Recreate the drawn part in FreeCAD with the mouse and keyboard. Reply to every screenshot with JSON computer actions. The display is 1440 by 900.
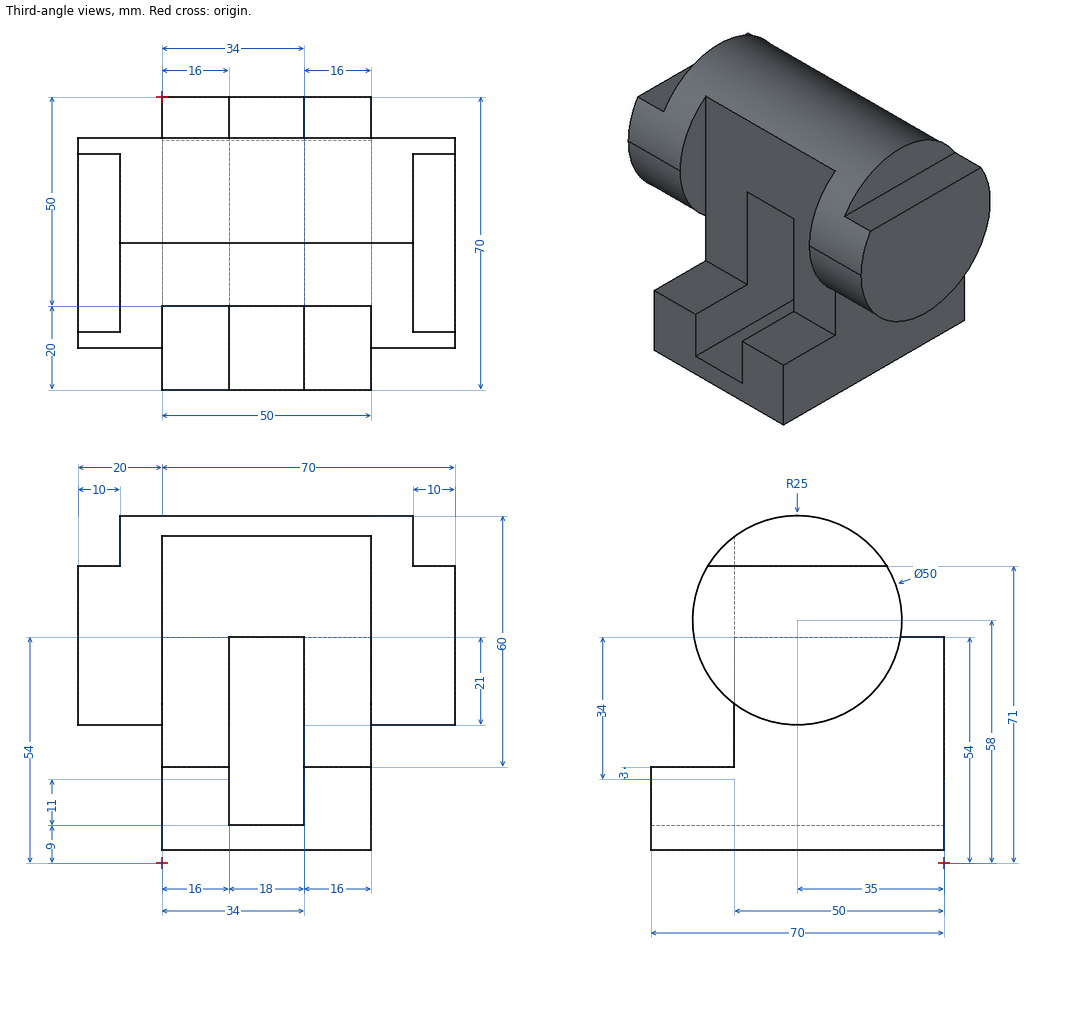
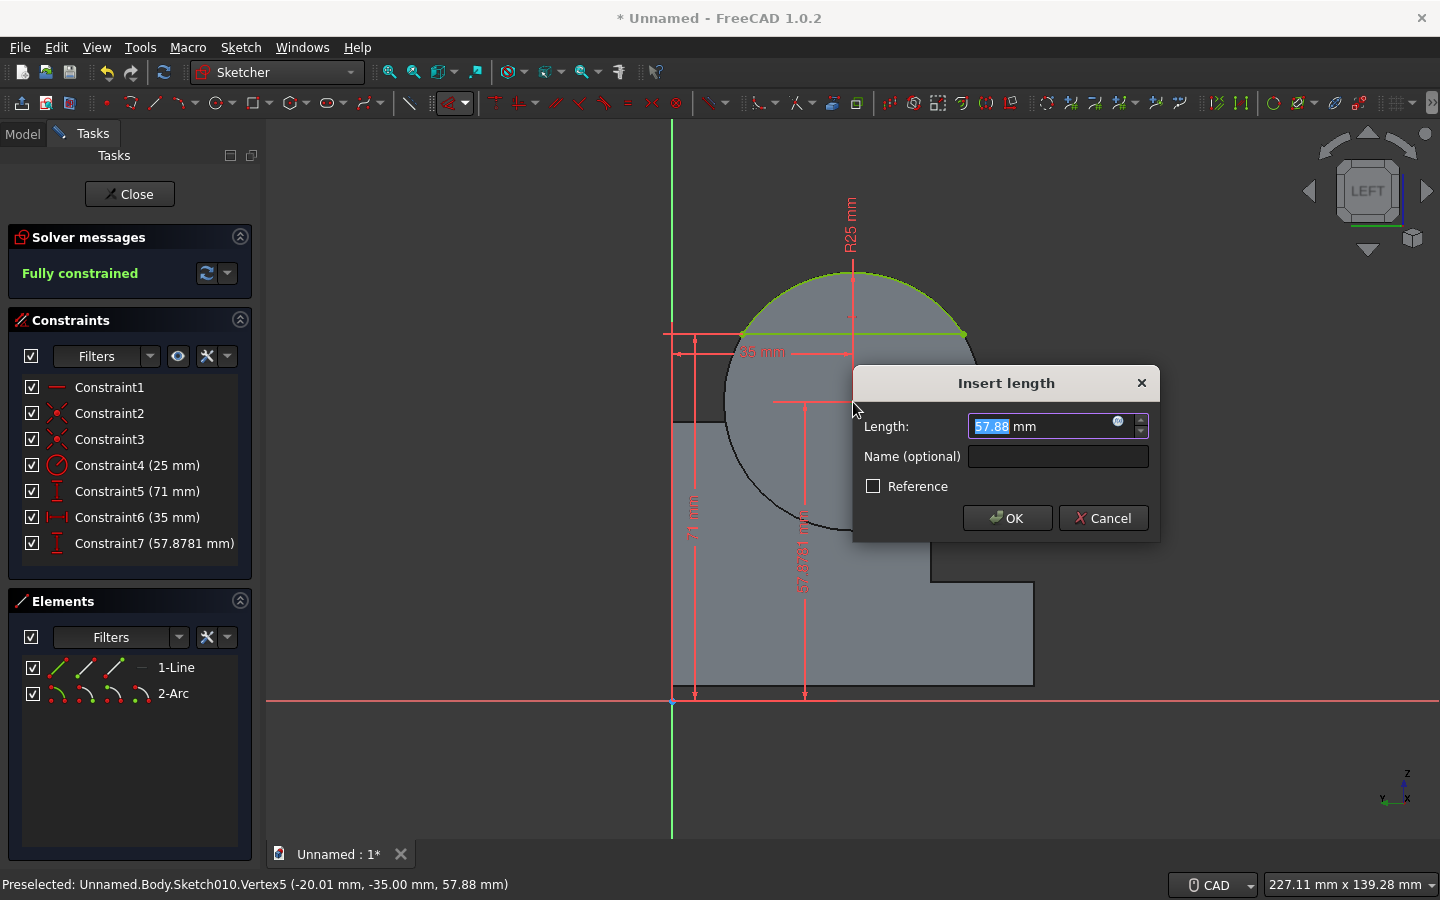
{"action": "type", "text": "58"}
{"action": "key", "text": "Return"}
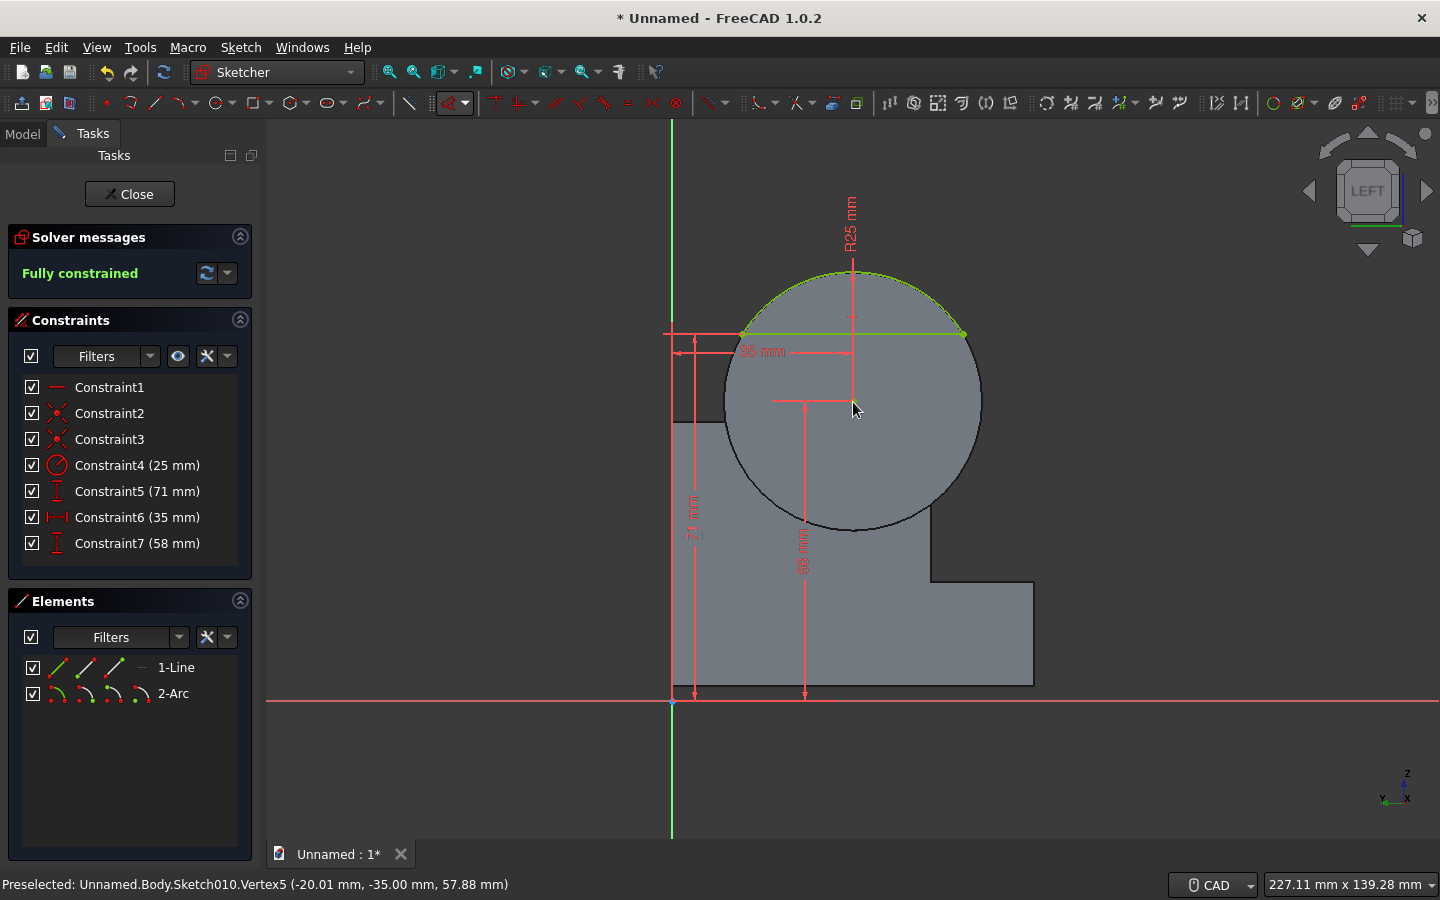
{"action": "left_click", "coordinate": [130, 194]}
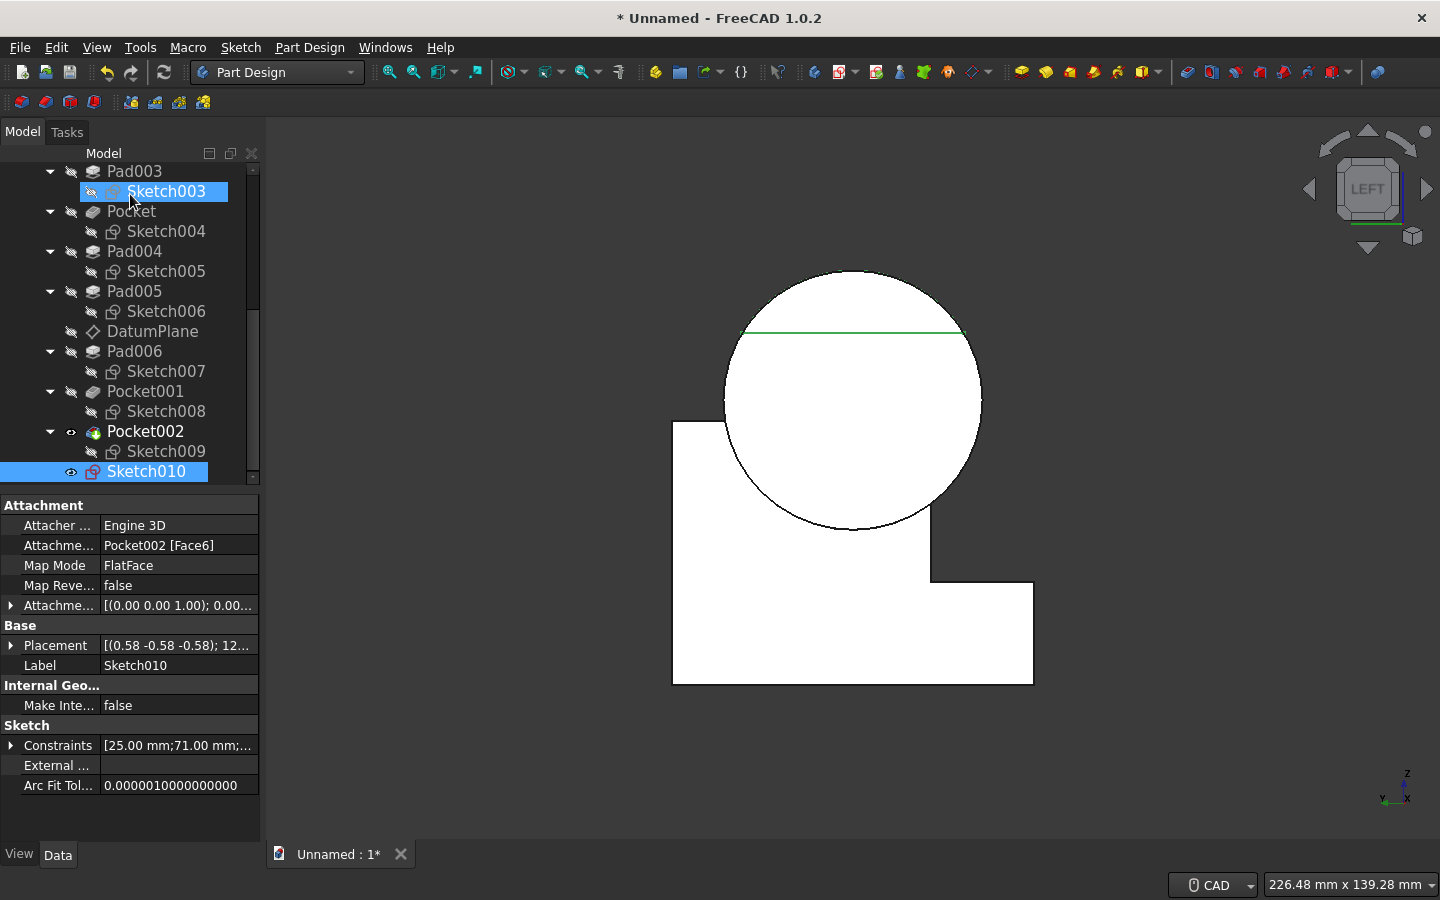
{"action": "left_click", "coordinate": [1188, 72]}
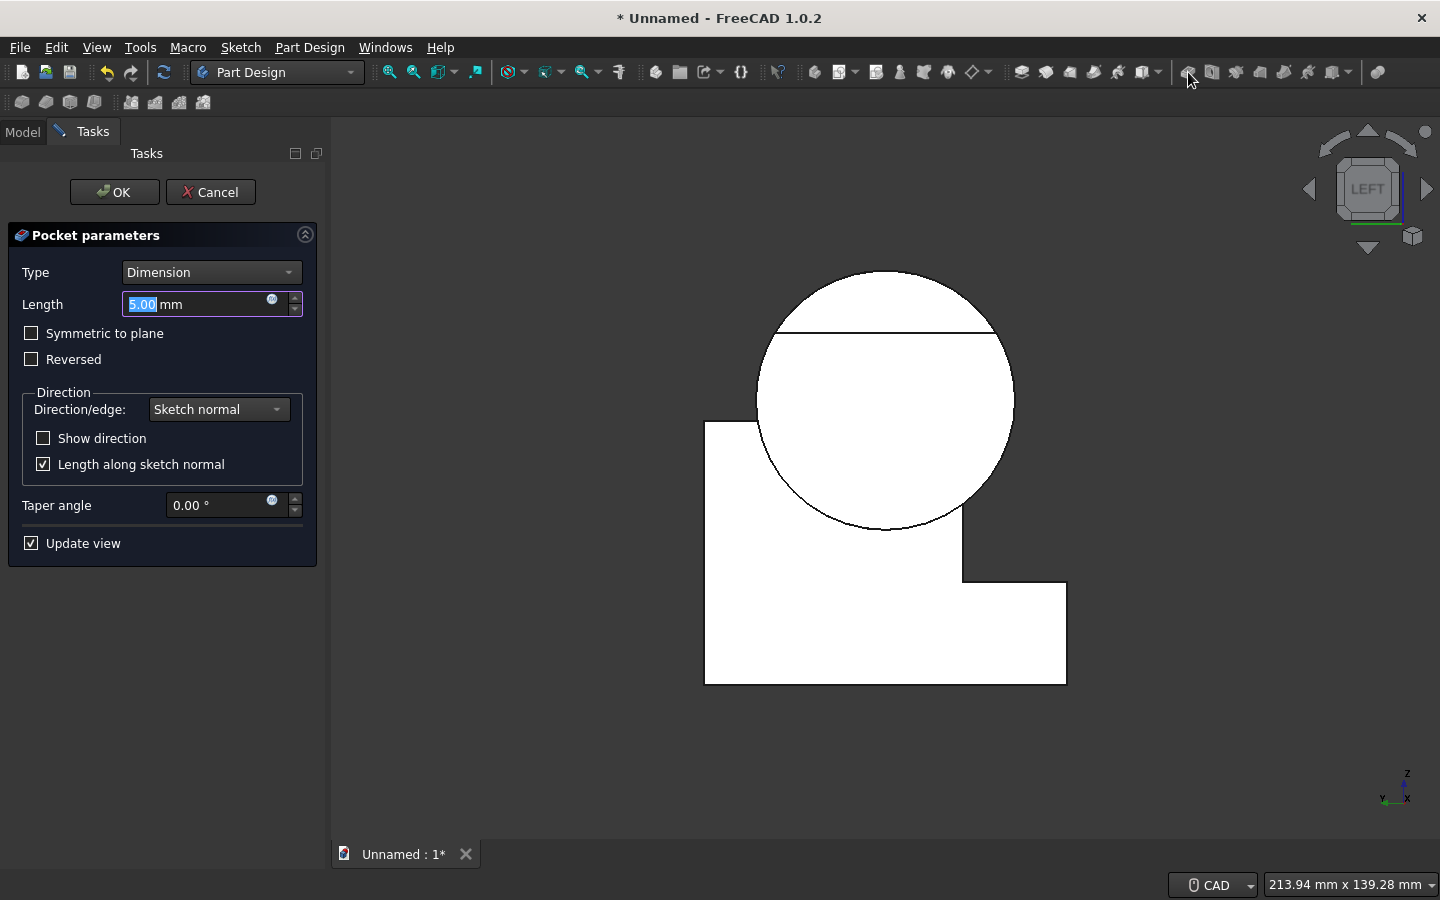
{"action": "type", "text": "10"}
{"action": "key", "text": "Tab"}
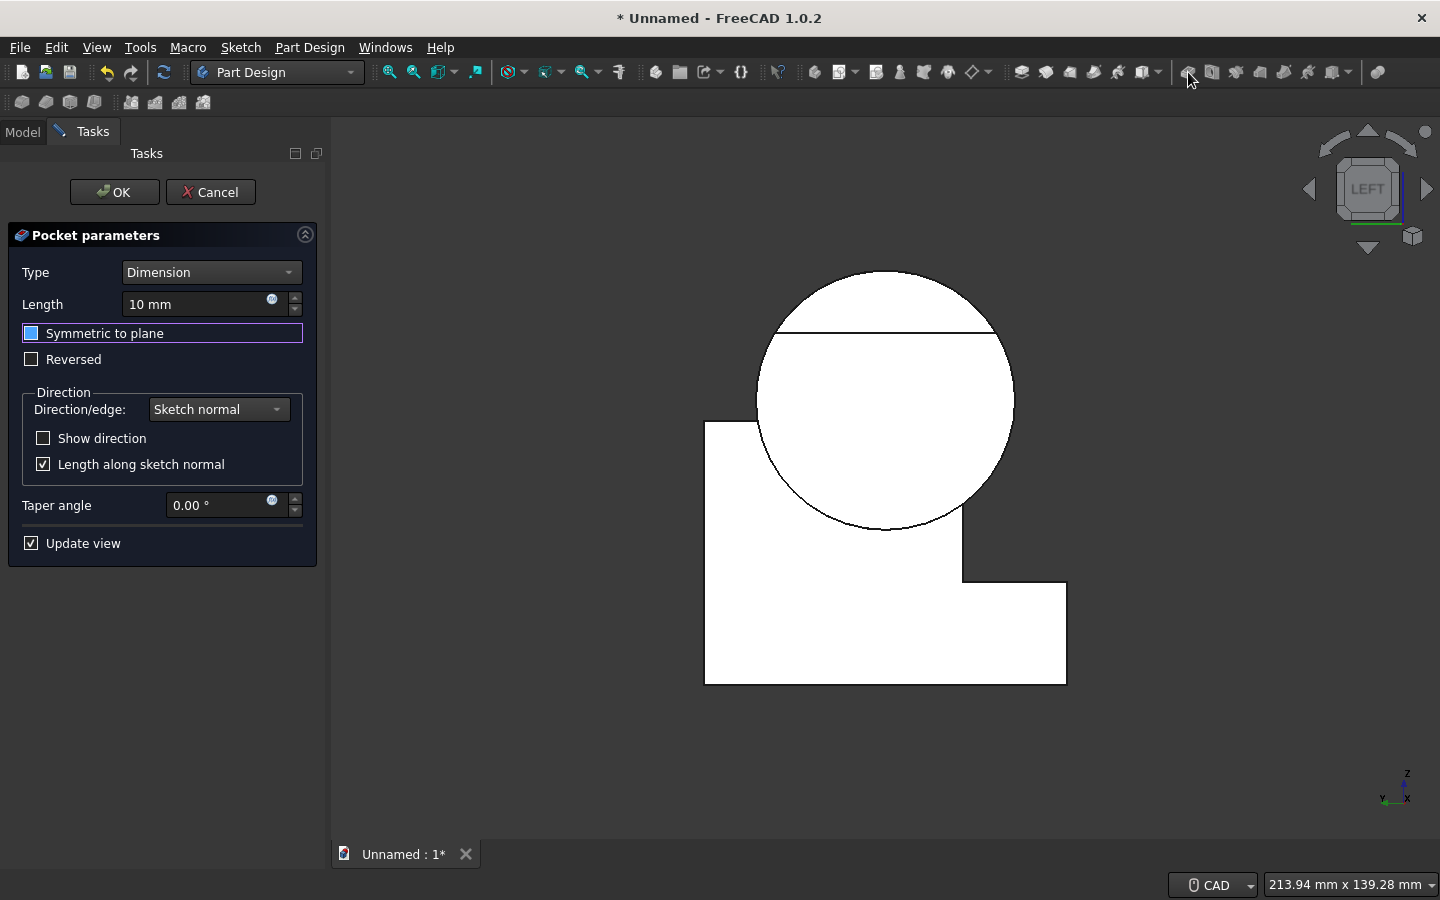
{"action": "left_click", "coordinate": [115, 192]}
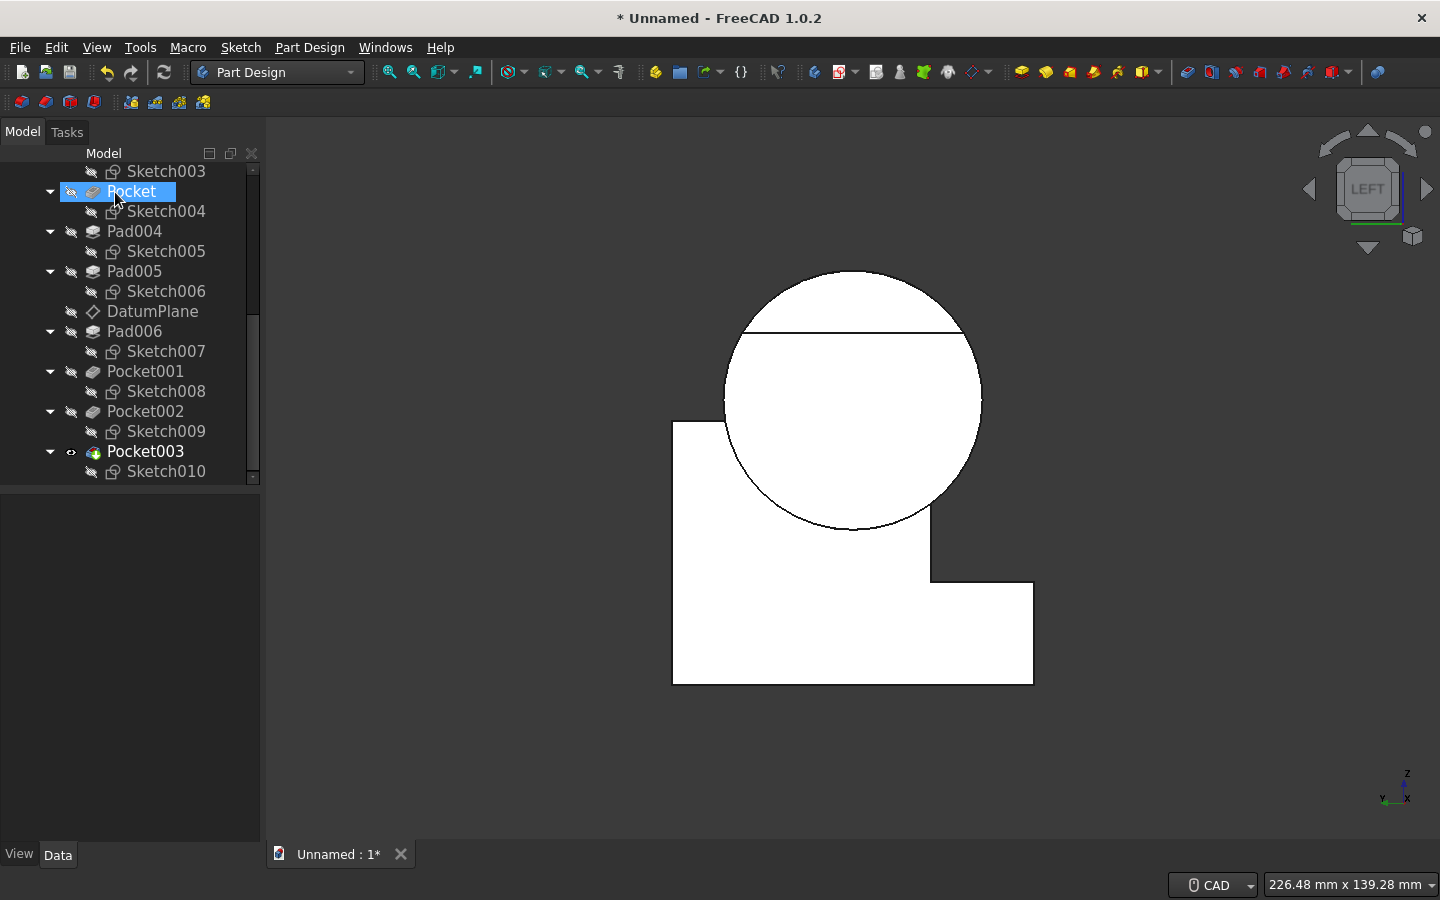
{"action": "scroll", "coordinate": [160, 327], "scroll_direction": "down", "scroll_amount": 3}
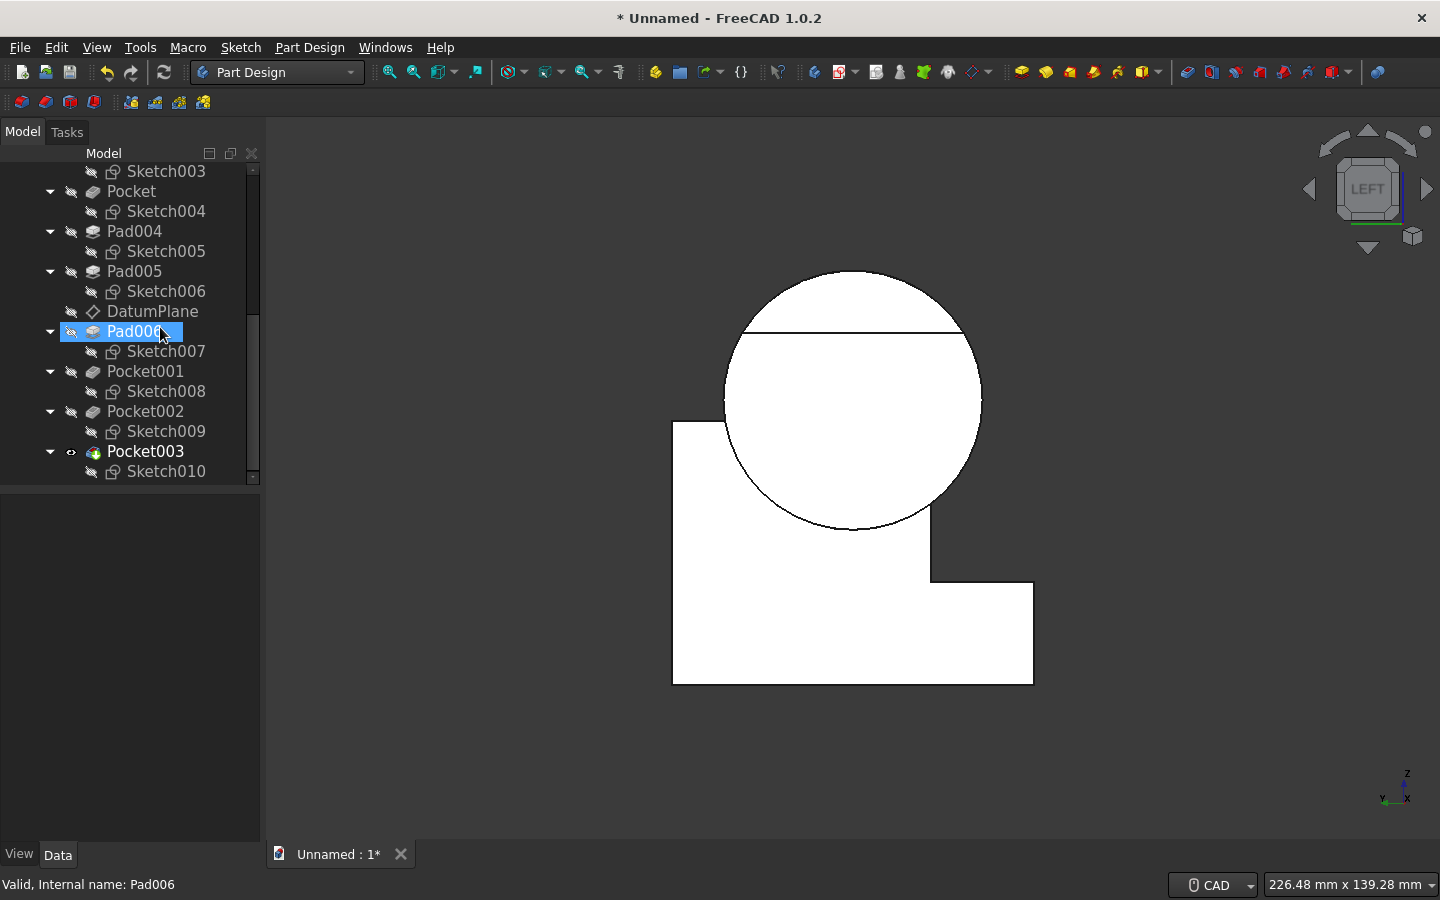
{"action": "scroll", "coordinate": [160, 327], "scroll_direction": "up", "scroll_amount": 15}